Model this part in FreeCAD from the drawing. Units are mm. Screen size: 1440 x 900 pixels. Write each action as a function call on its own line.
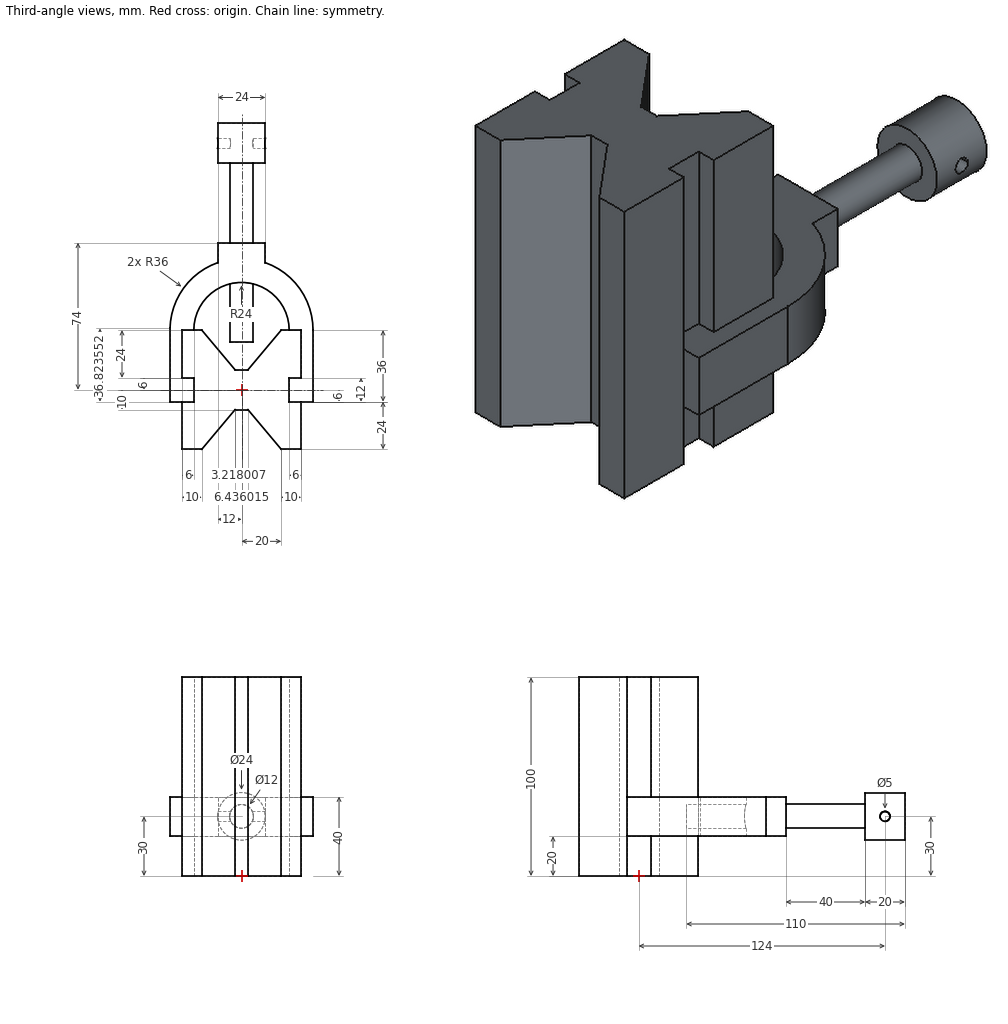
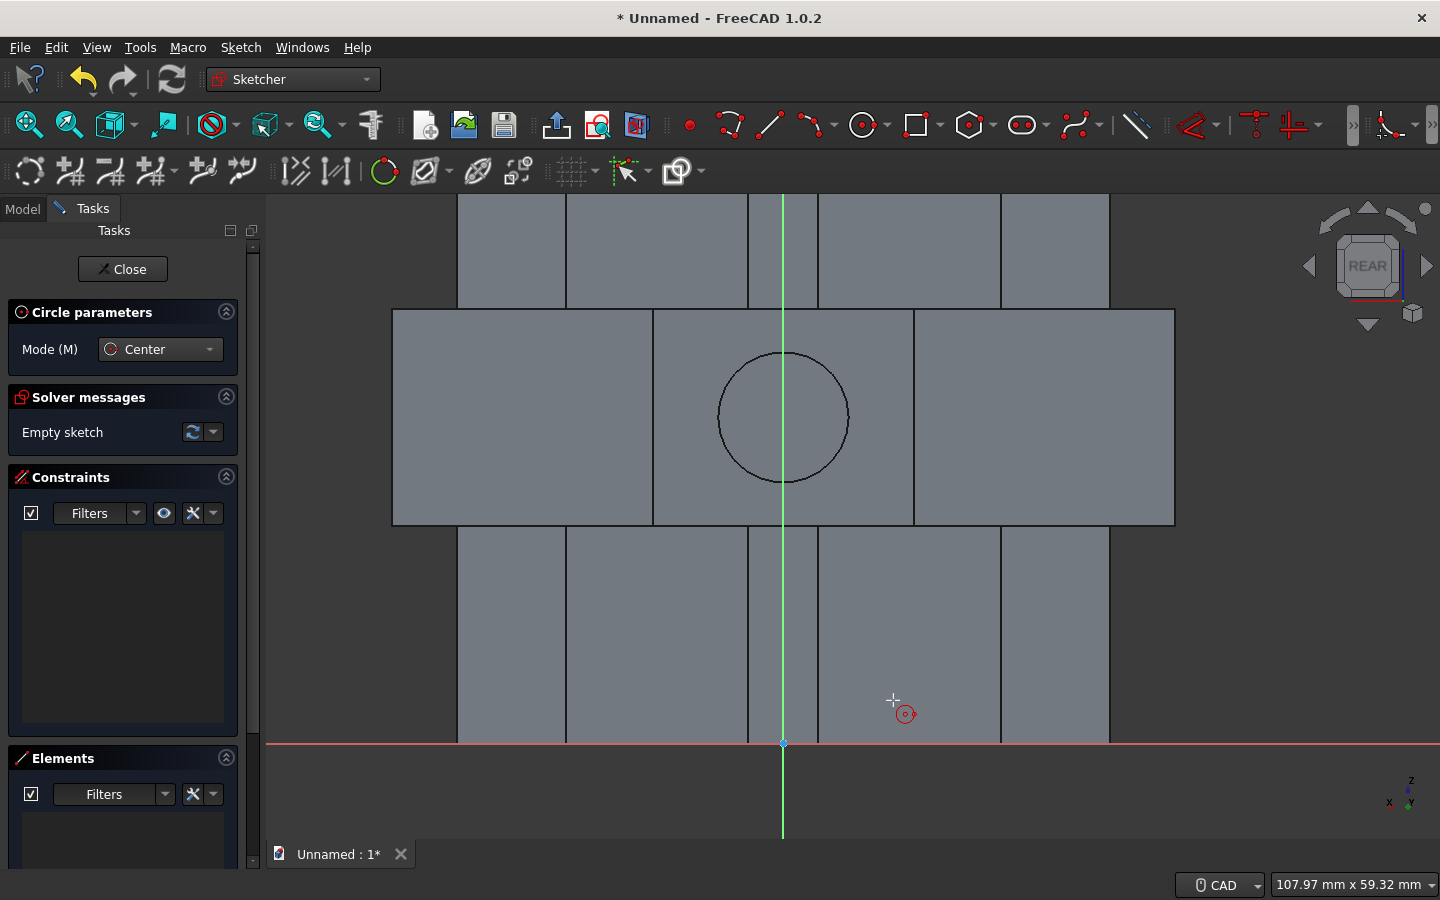
click(783, 417)
move(876, 325)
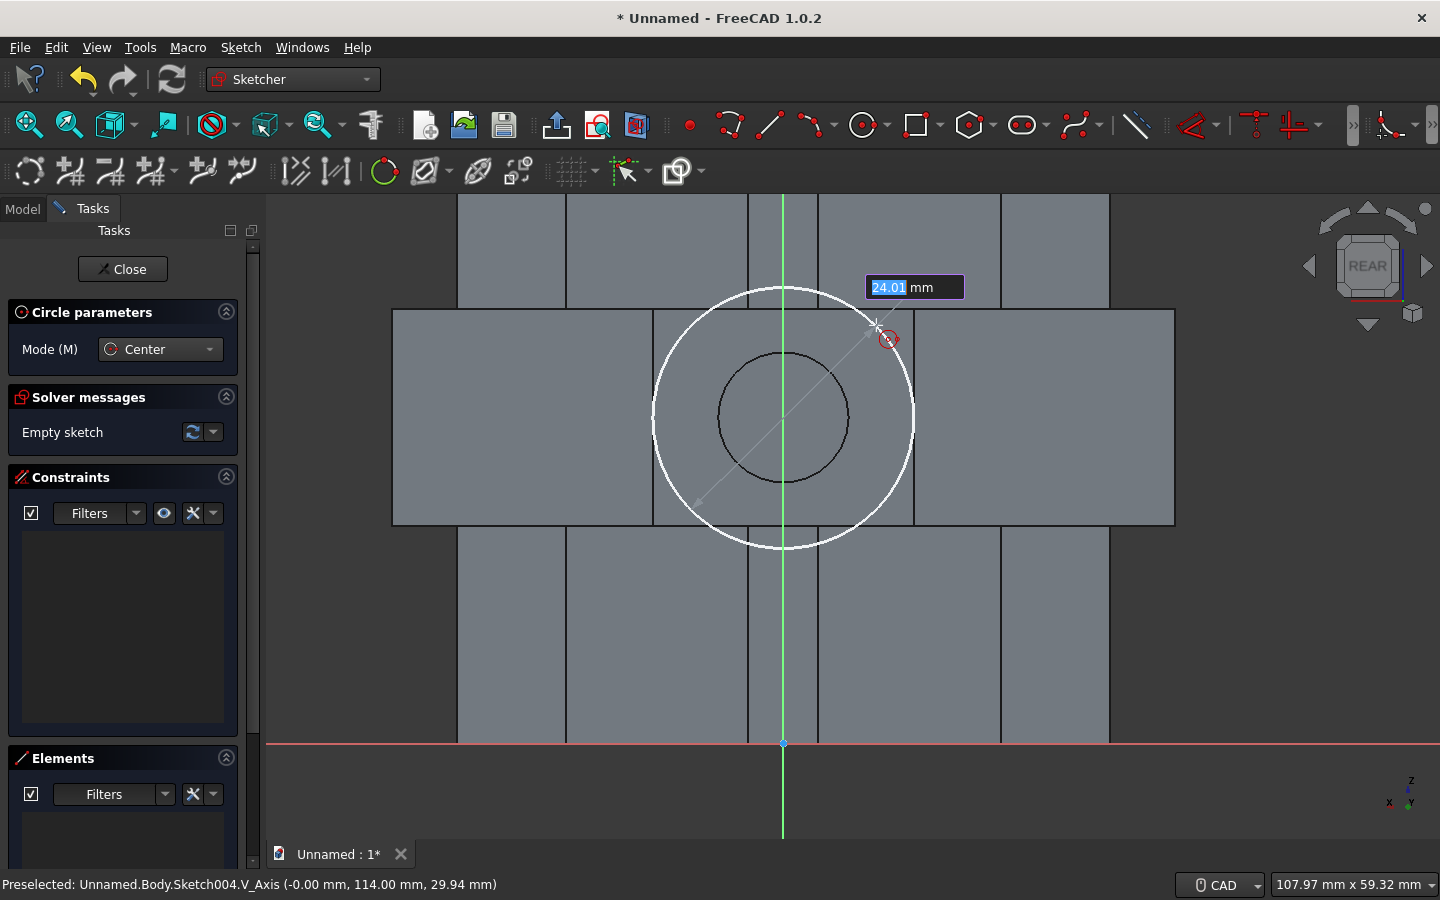
text(24)
key(Return)
key(Escape)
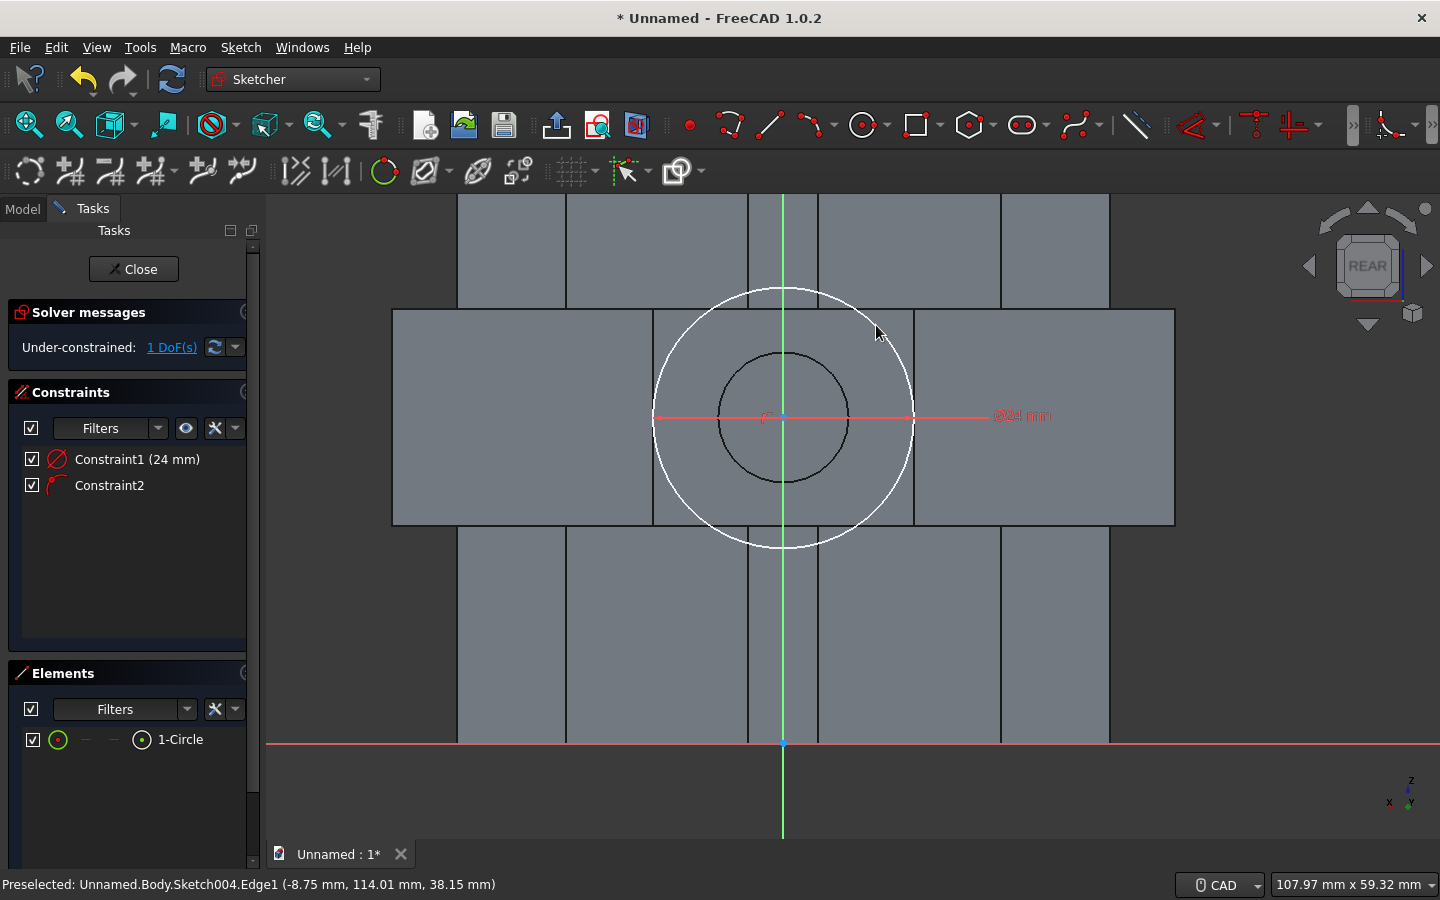
key(d)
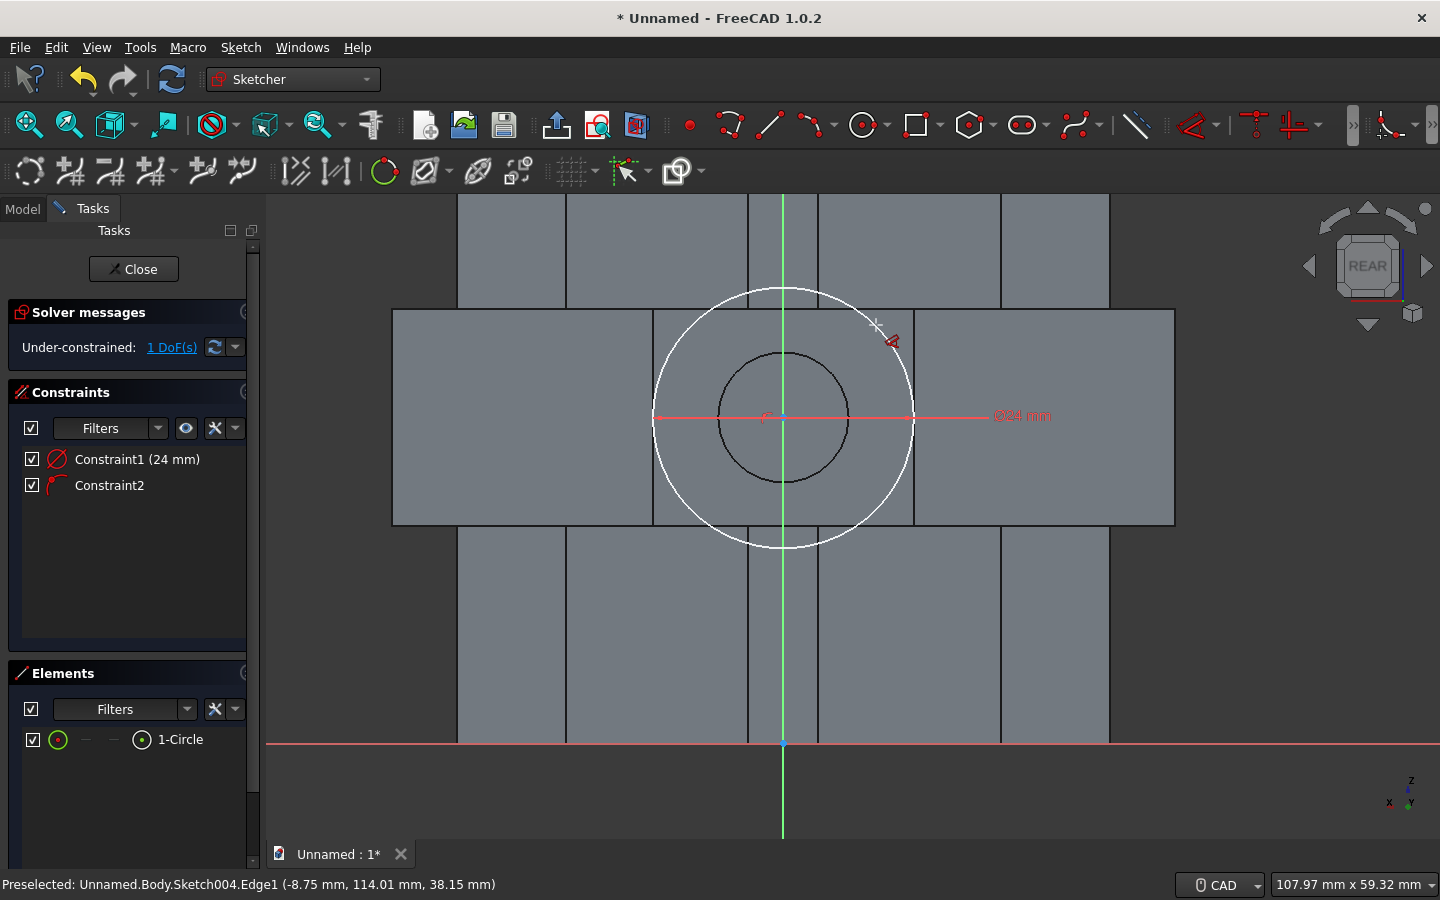
click(783, 418)
click(817, 581)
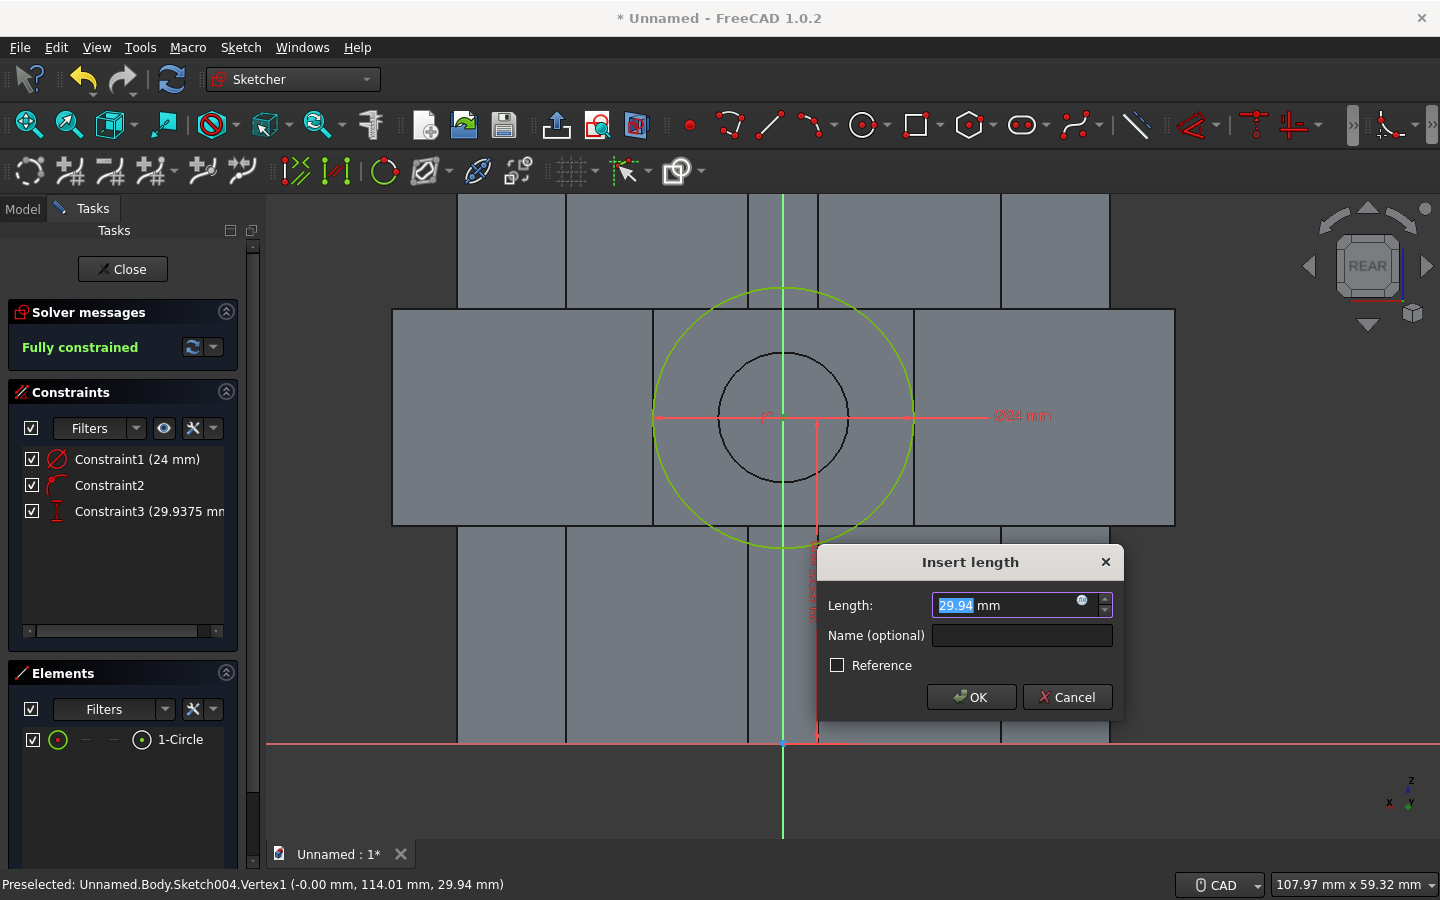
text(30)
key(Return)
key(Escape)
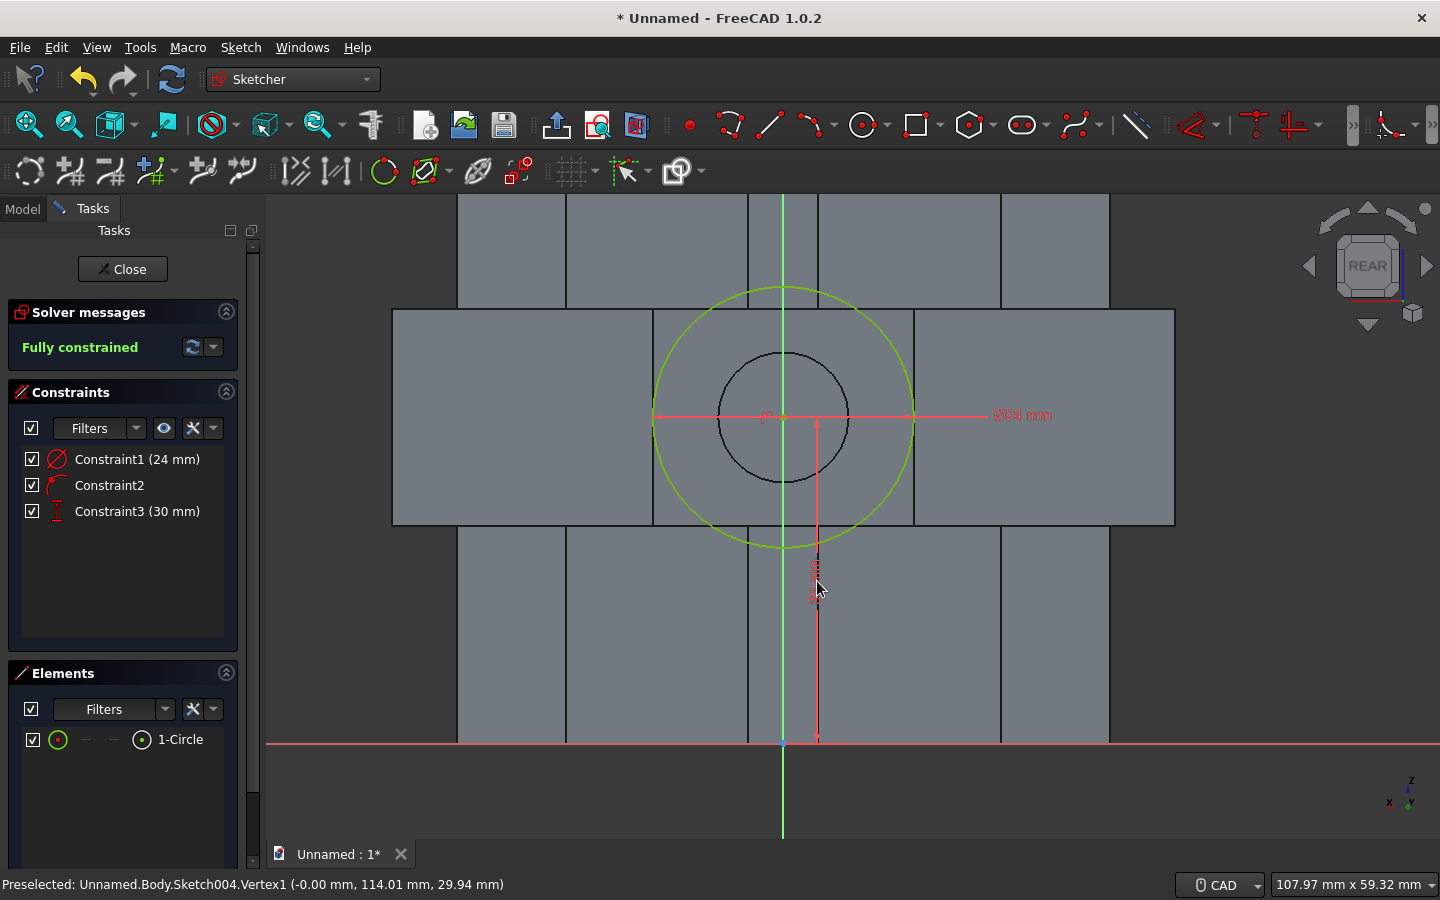
click(123, 269)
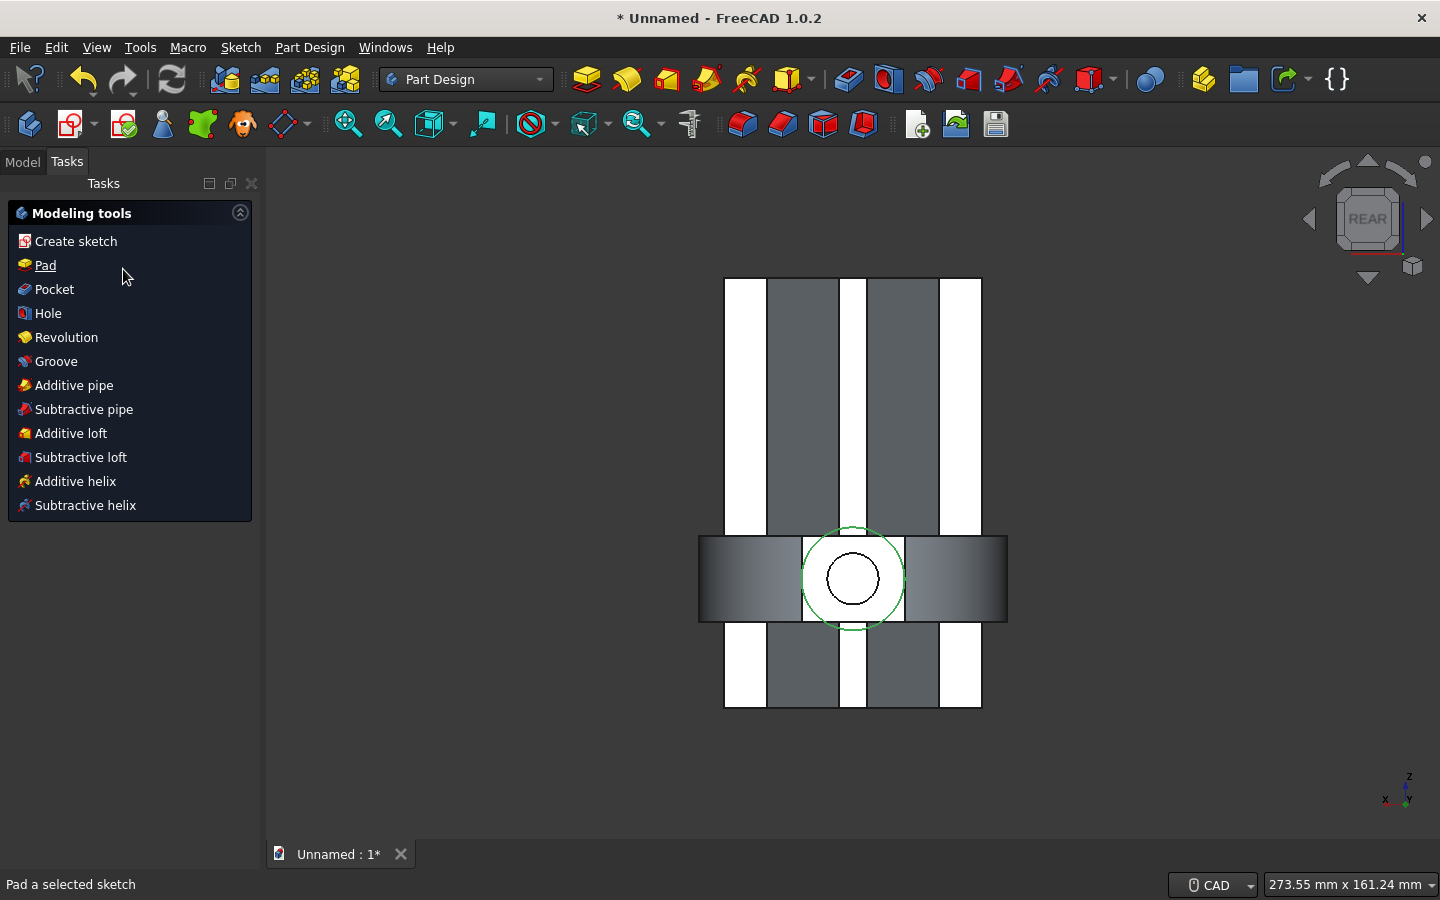
click(588, 80)